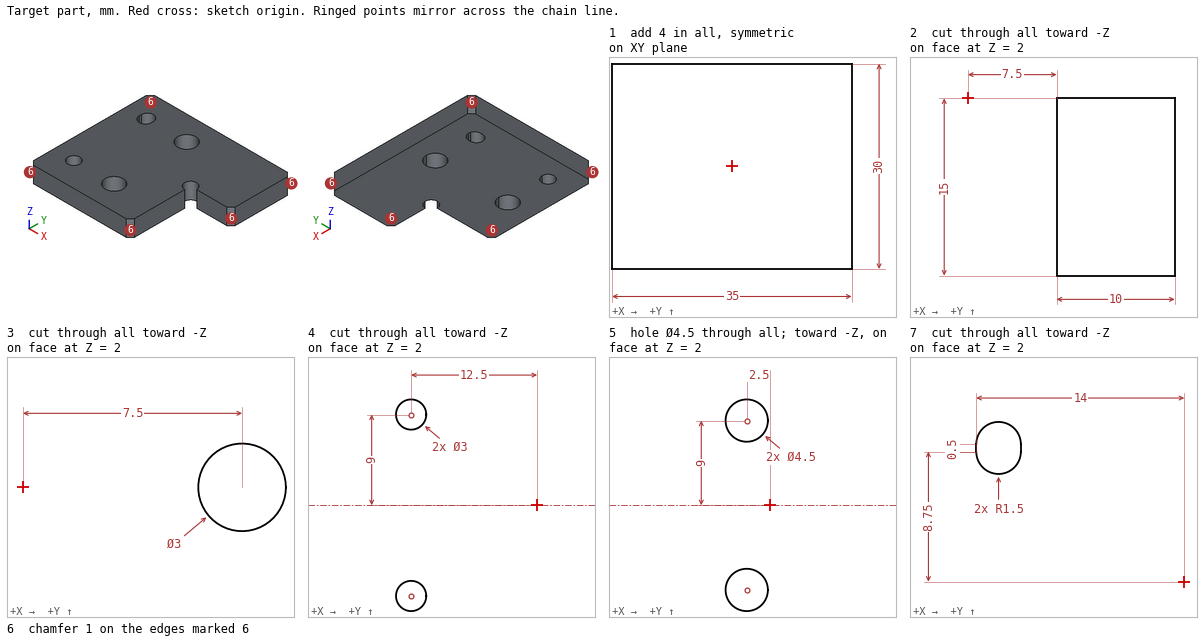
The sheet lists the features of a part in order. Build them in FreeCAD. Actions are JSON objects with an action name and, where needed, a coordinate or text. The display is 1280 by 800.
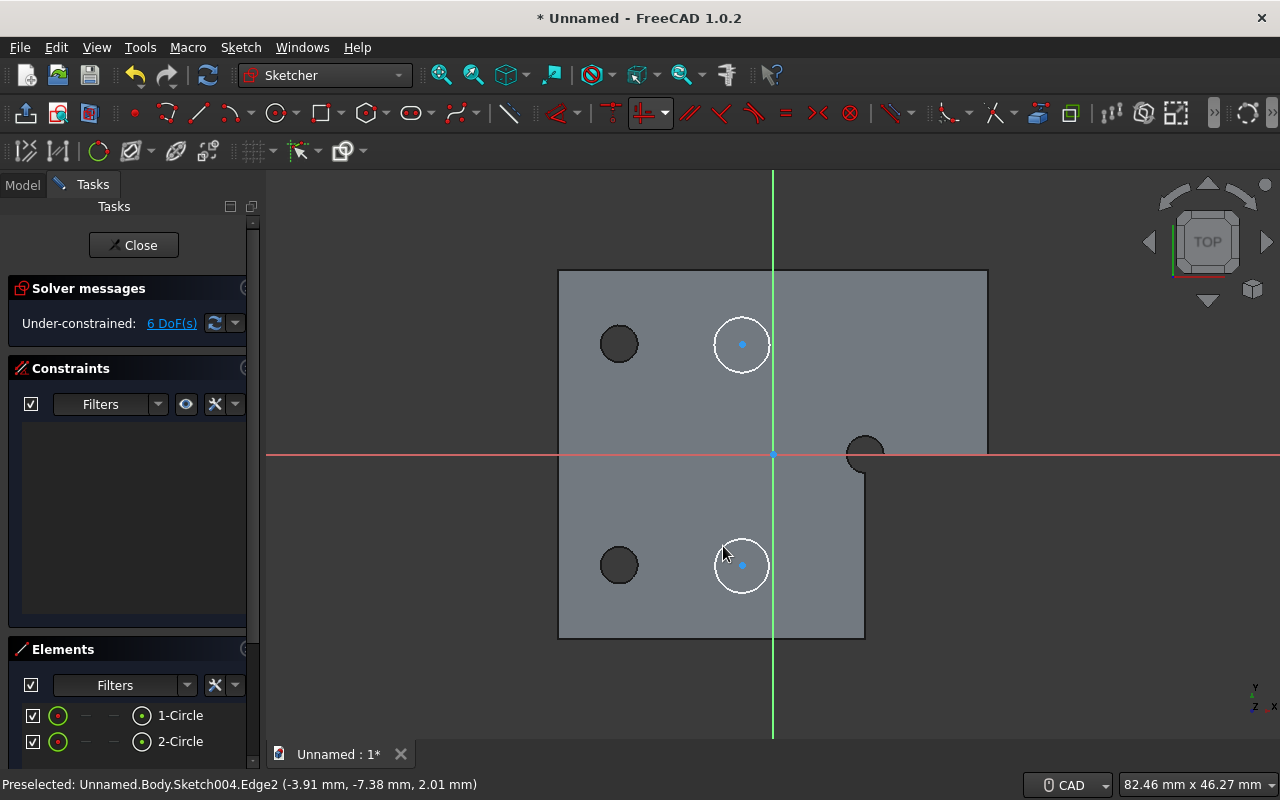
{"action": "left_click", "coordinate": [761, 325]}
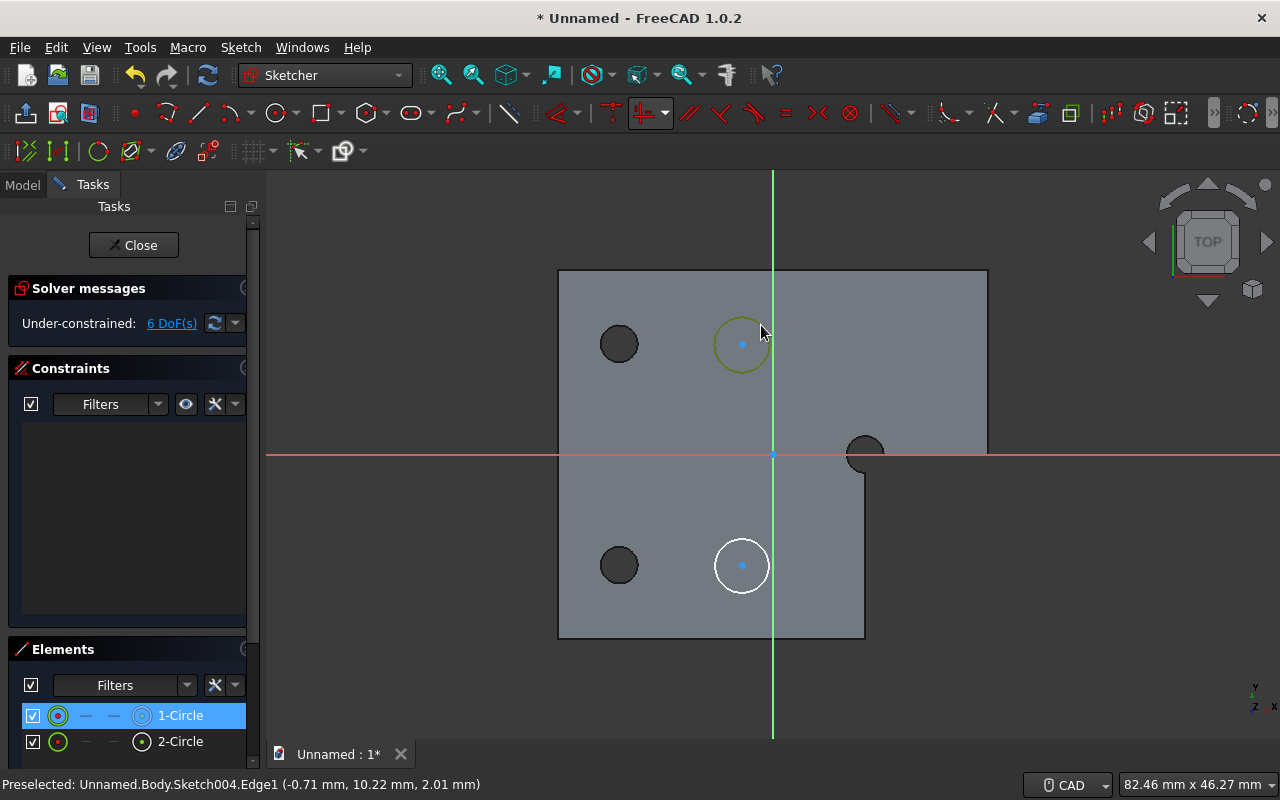
{"action": "left_click", "coordinate": [761, 547]}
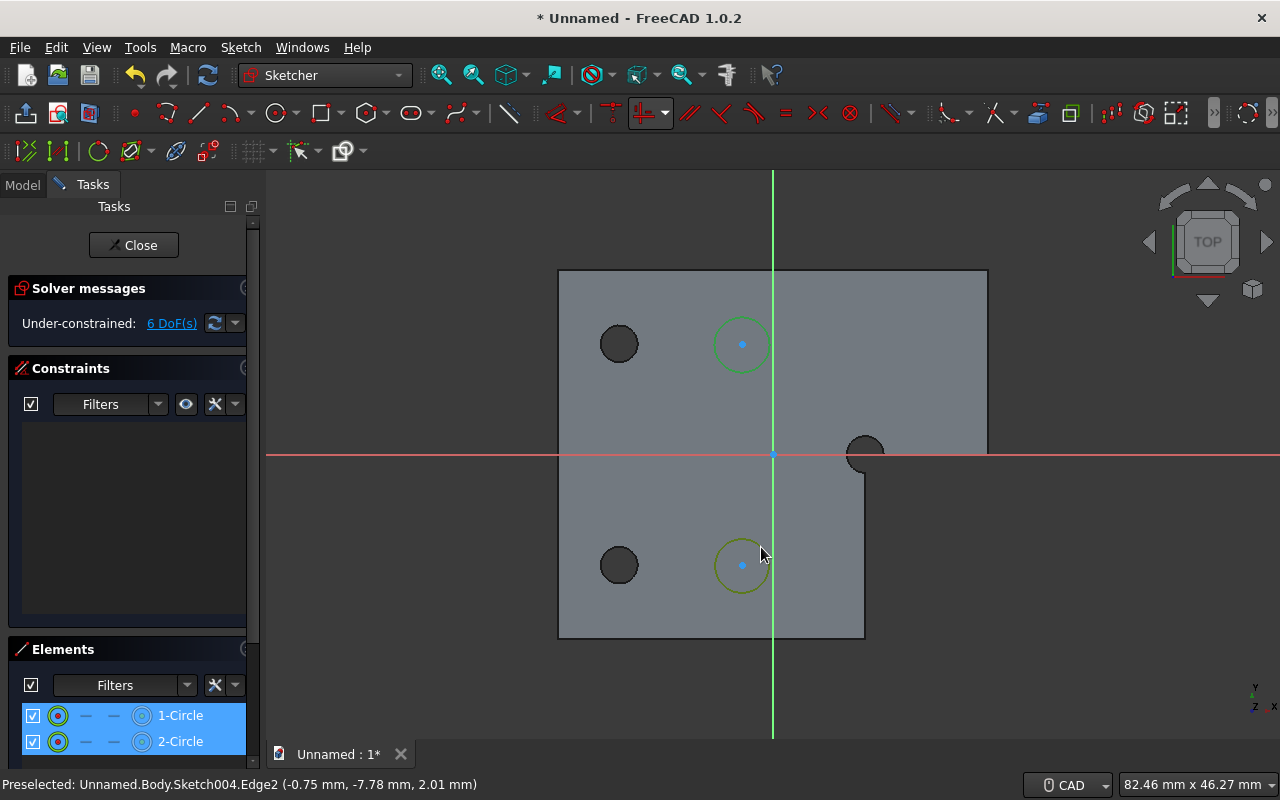
{"action": "key", "text": "e"}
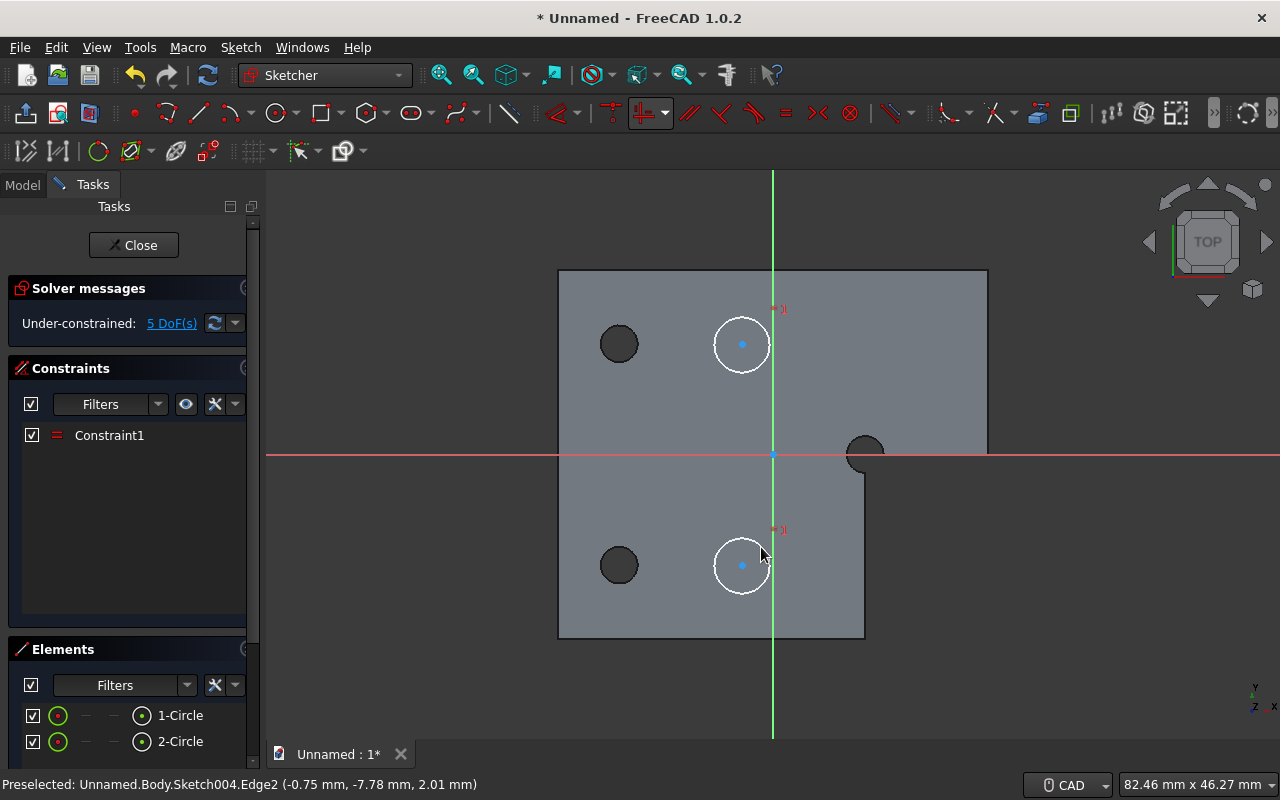
{"action": "left_click", "coordinate": [742, 345]}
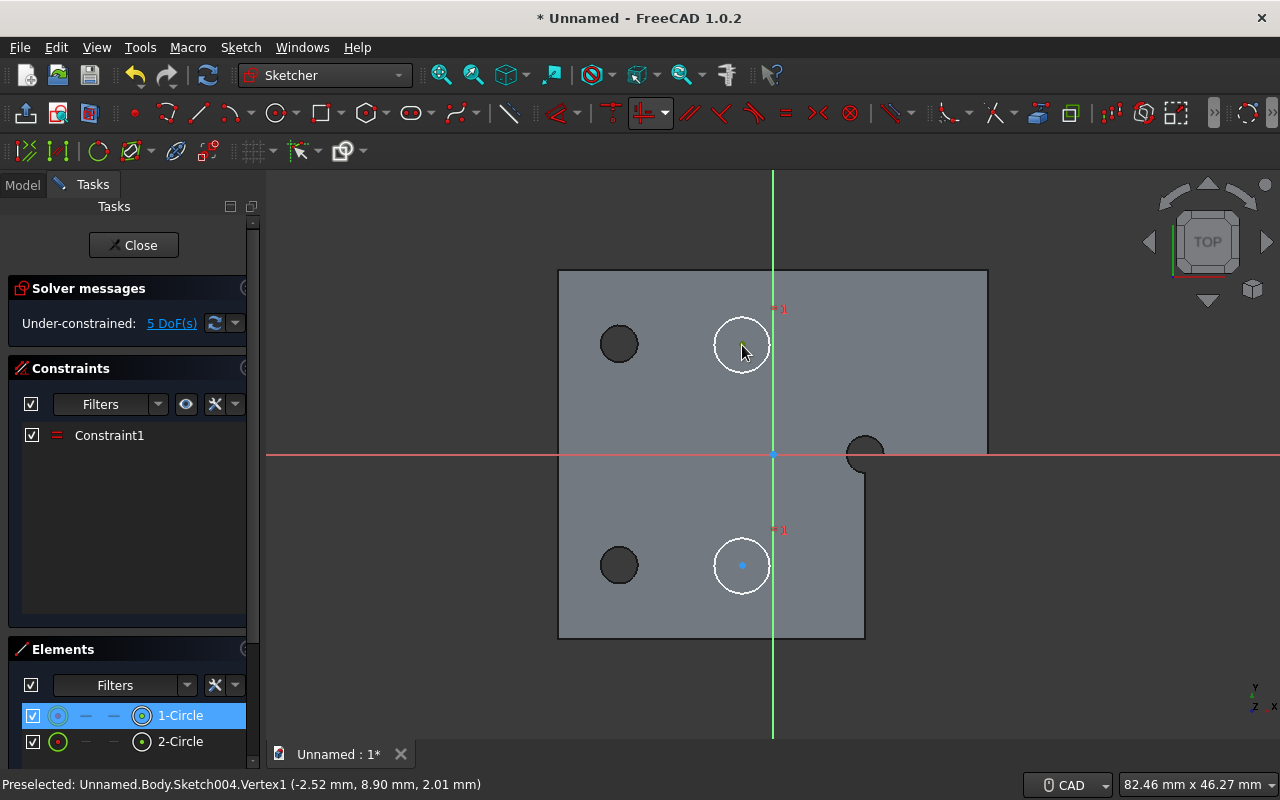
{"action": "left_click", "coordinate": [742, 566]}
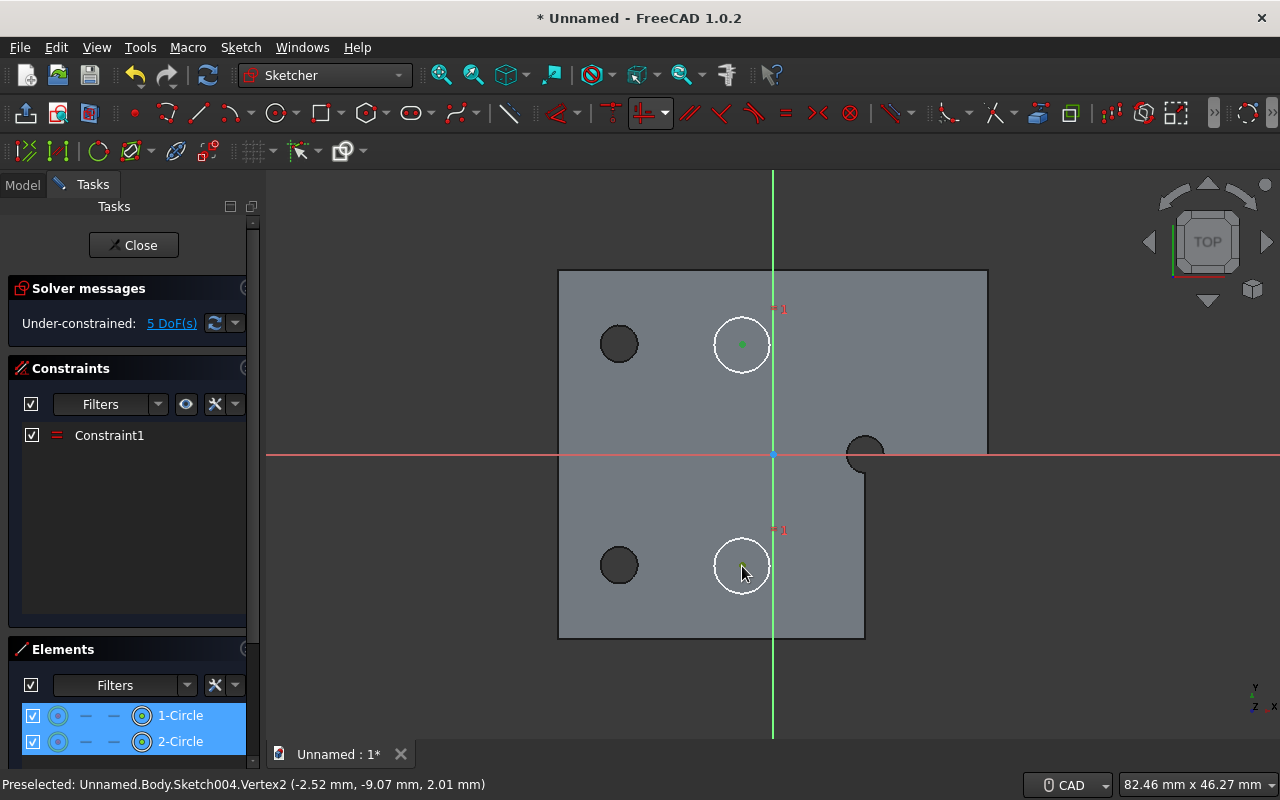
{"action": "left_click", "coordinate": [353, 454]}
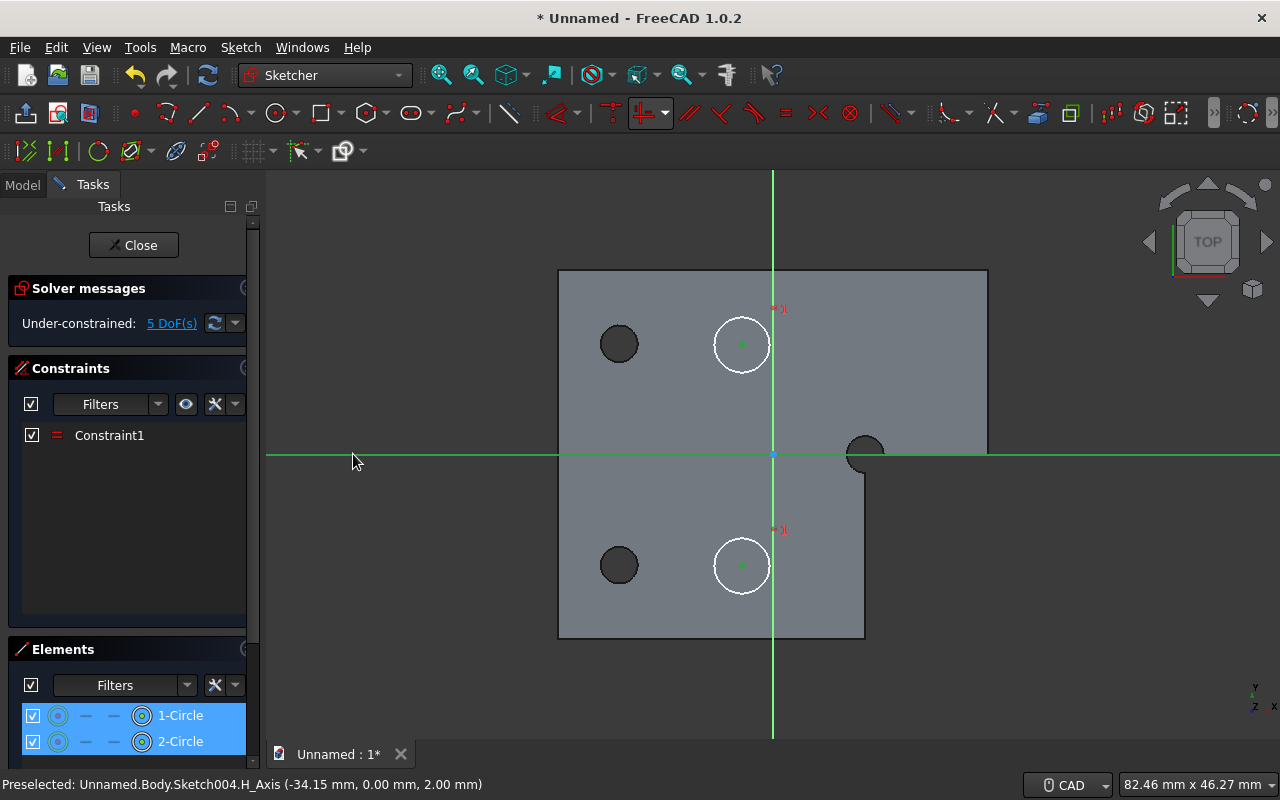
{"action": "left_click", "coordinate": [818, 114]}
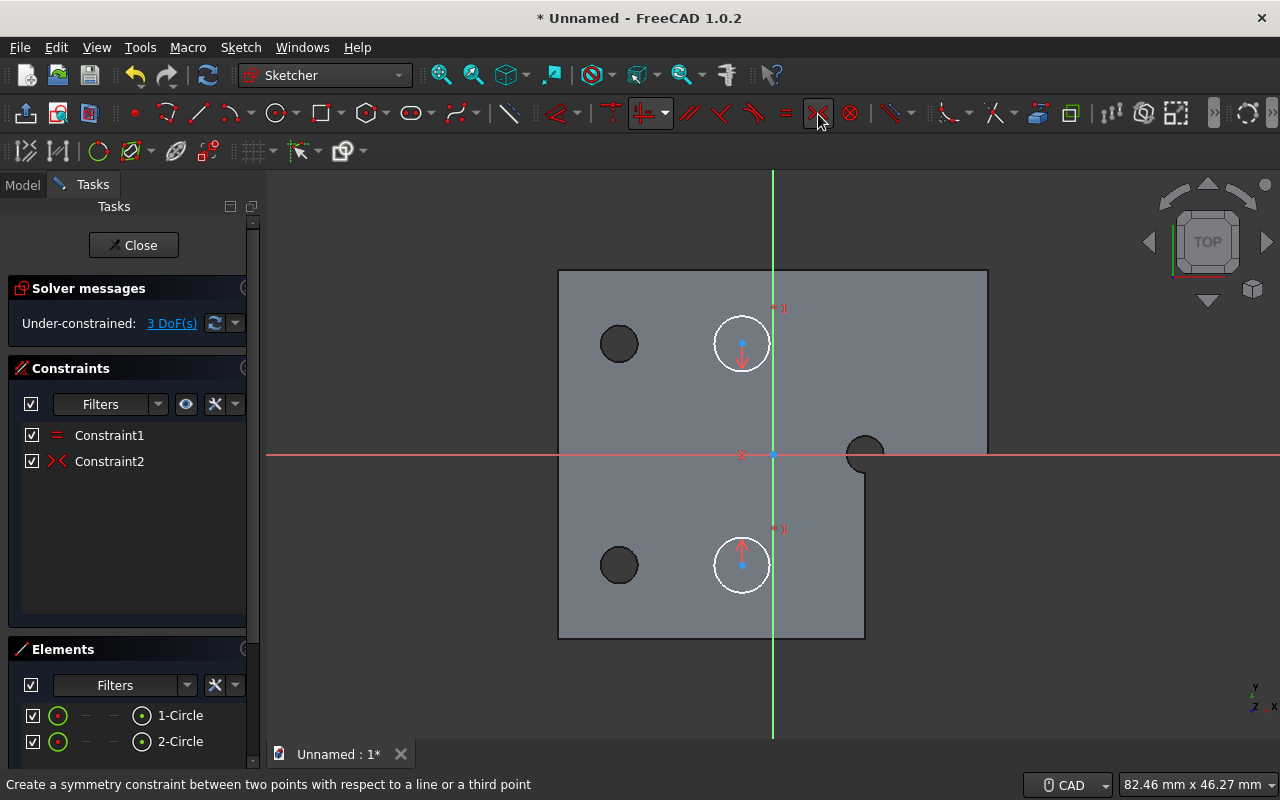
{"action": "key", "text": "d"}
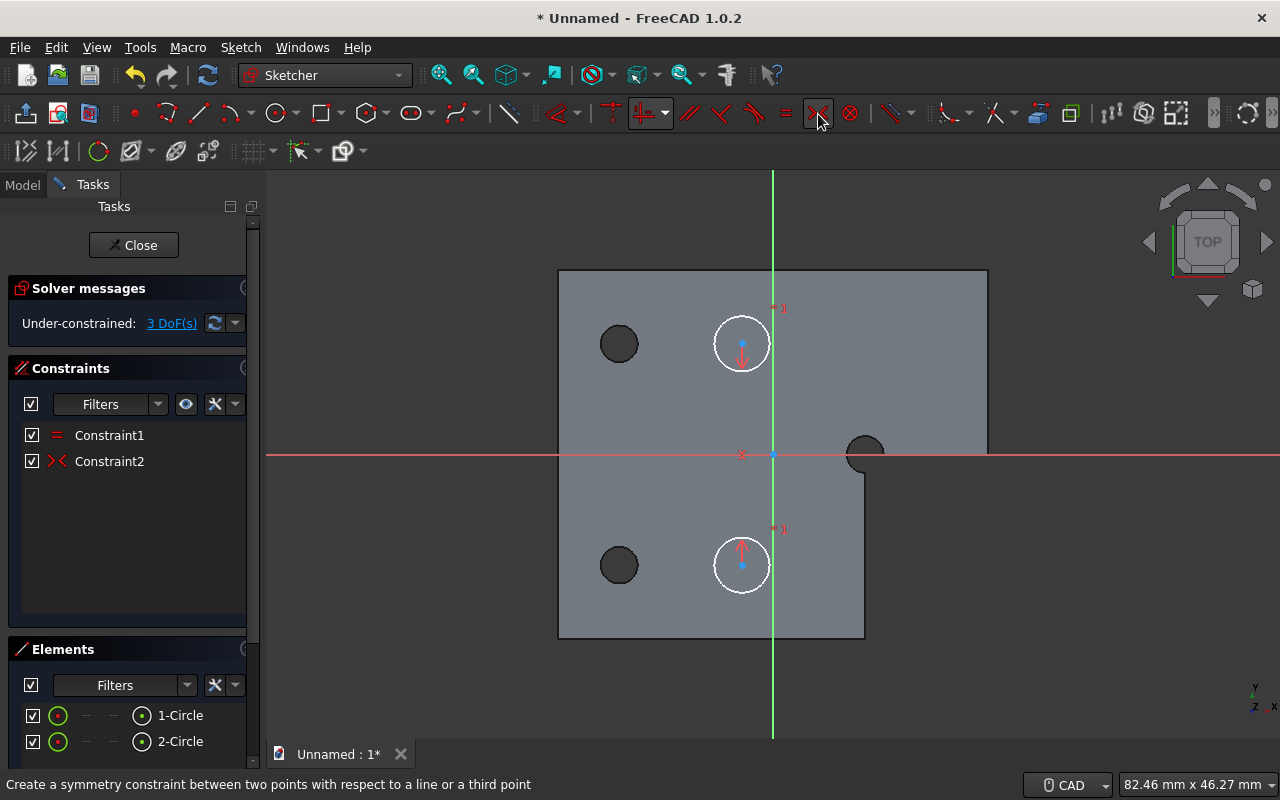
{"action": "left_click", "coordinate": [761, 324]}
{"action": "left_click", "coordinate": [799, 326]}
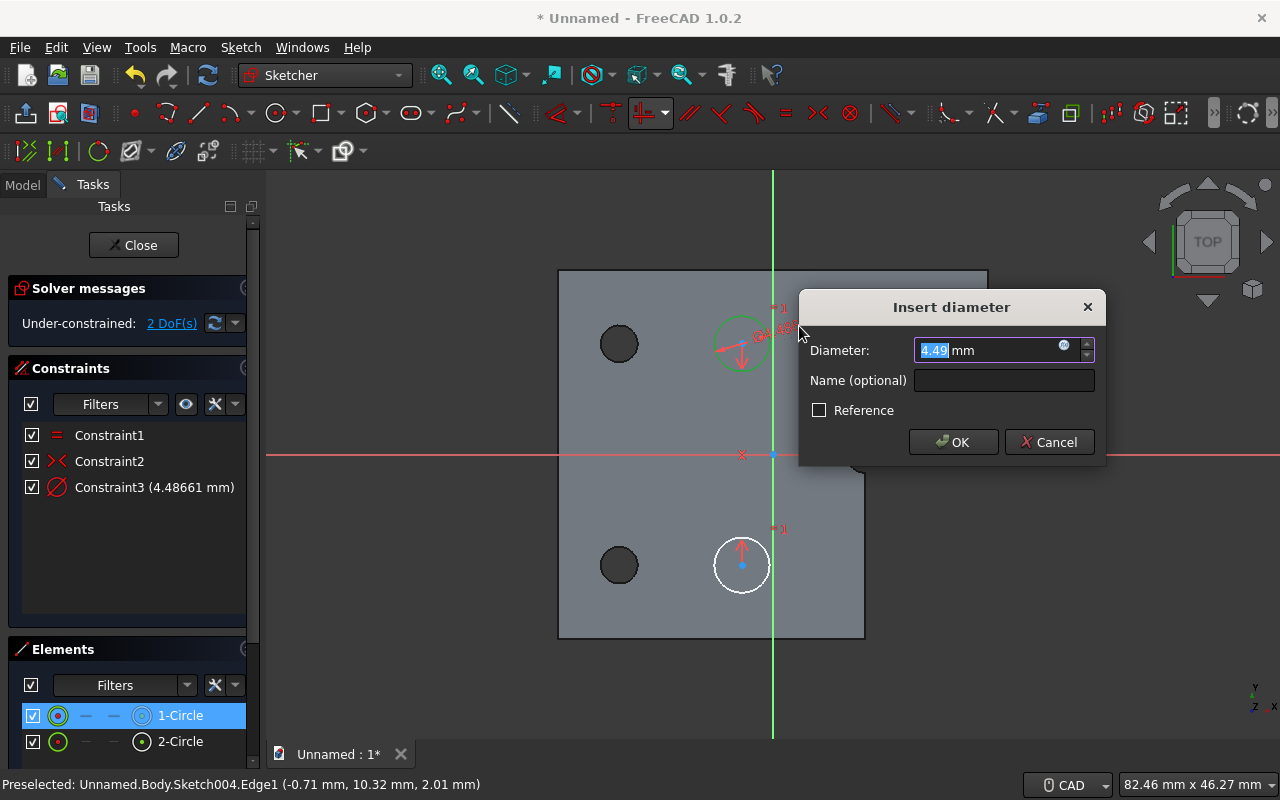
{"action": "type", "text": "4.5"}
{"action": "key", "text": "Return"}